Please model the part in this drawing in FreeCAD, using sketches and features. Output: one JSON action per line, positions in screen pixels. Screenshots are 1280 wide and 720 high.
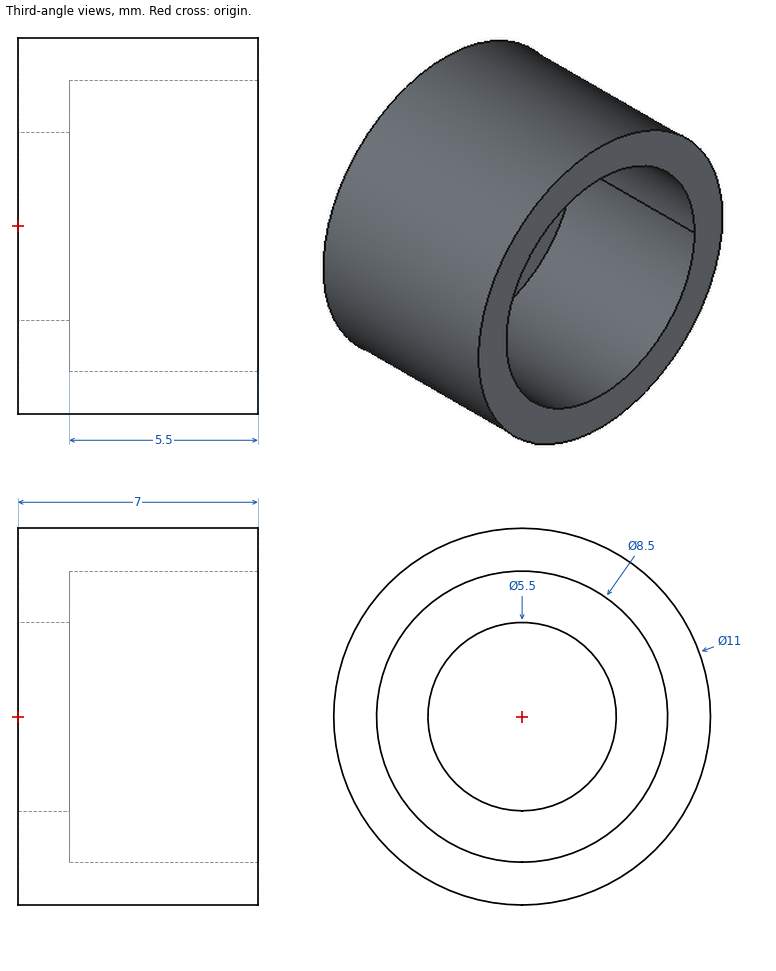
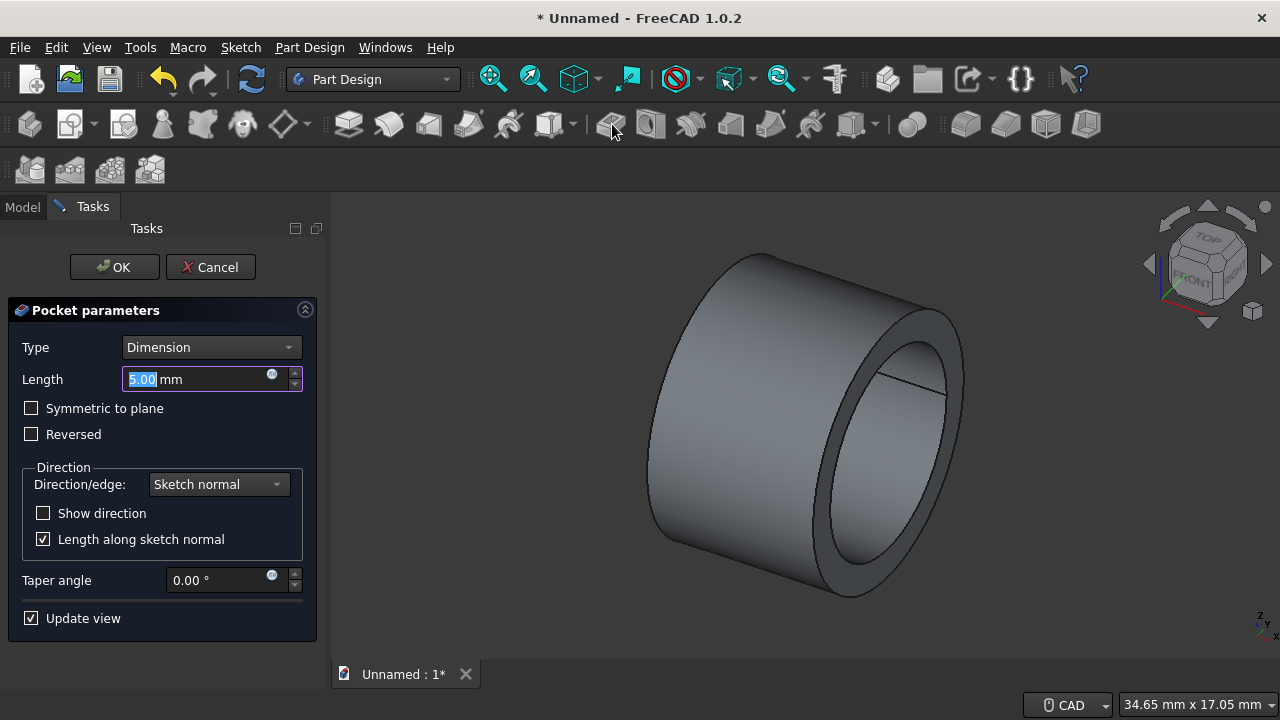
{"action": "type", "text": "5.5"}
{"action": "key", "text": "Tab"}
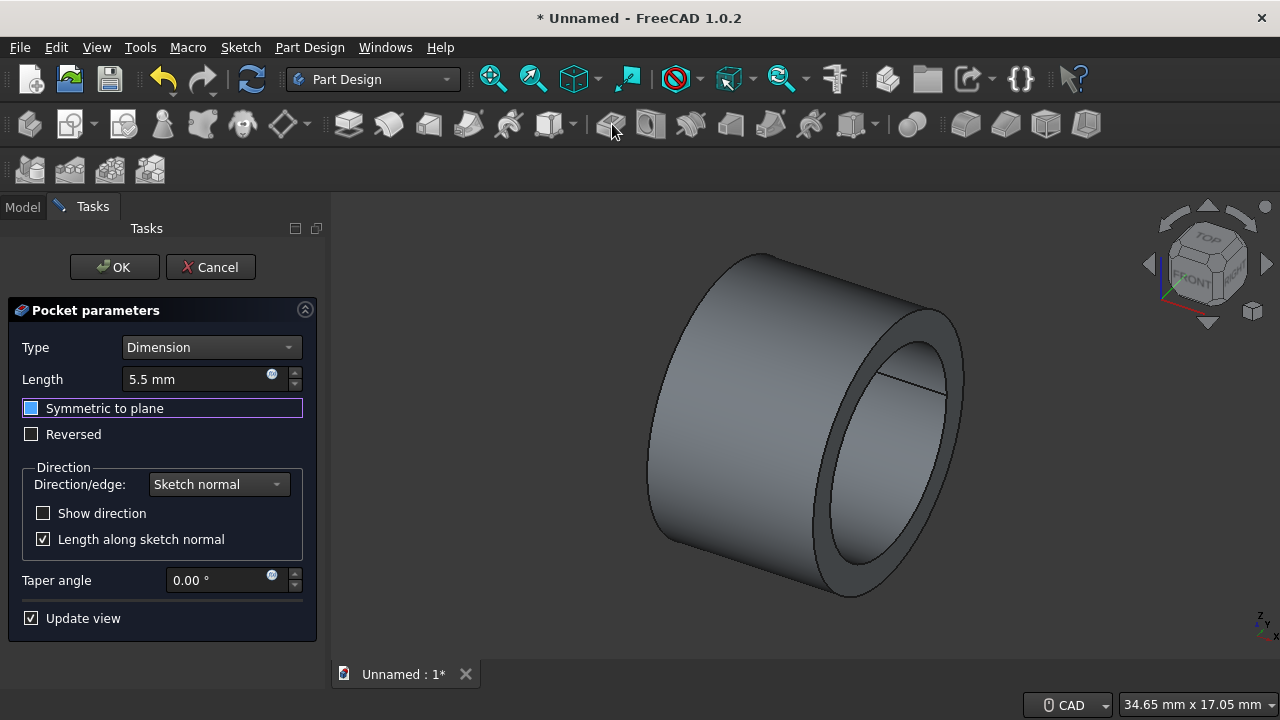
{"action": "left_click", "coordinate": [115, 267]}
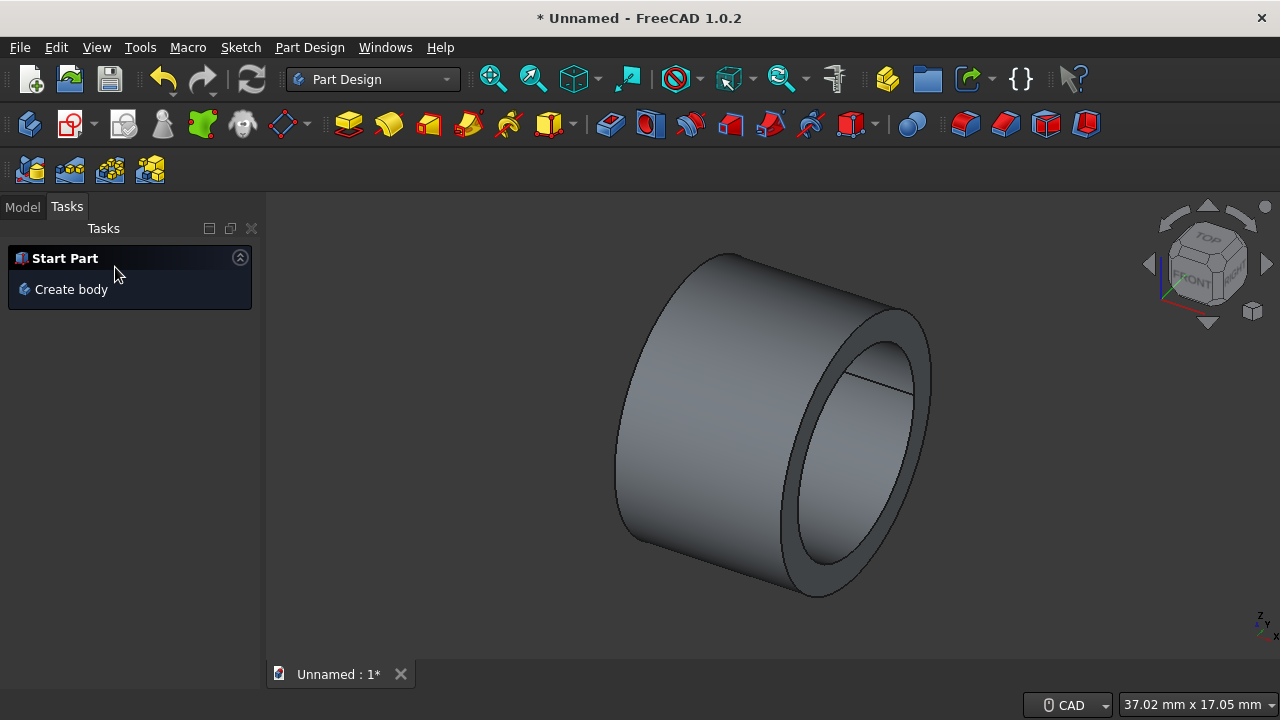
{"action": "key", "text": "0"}